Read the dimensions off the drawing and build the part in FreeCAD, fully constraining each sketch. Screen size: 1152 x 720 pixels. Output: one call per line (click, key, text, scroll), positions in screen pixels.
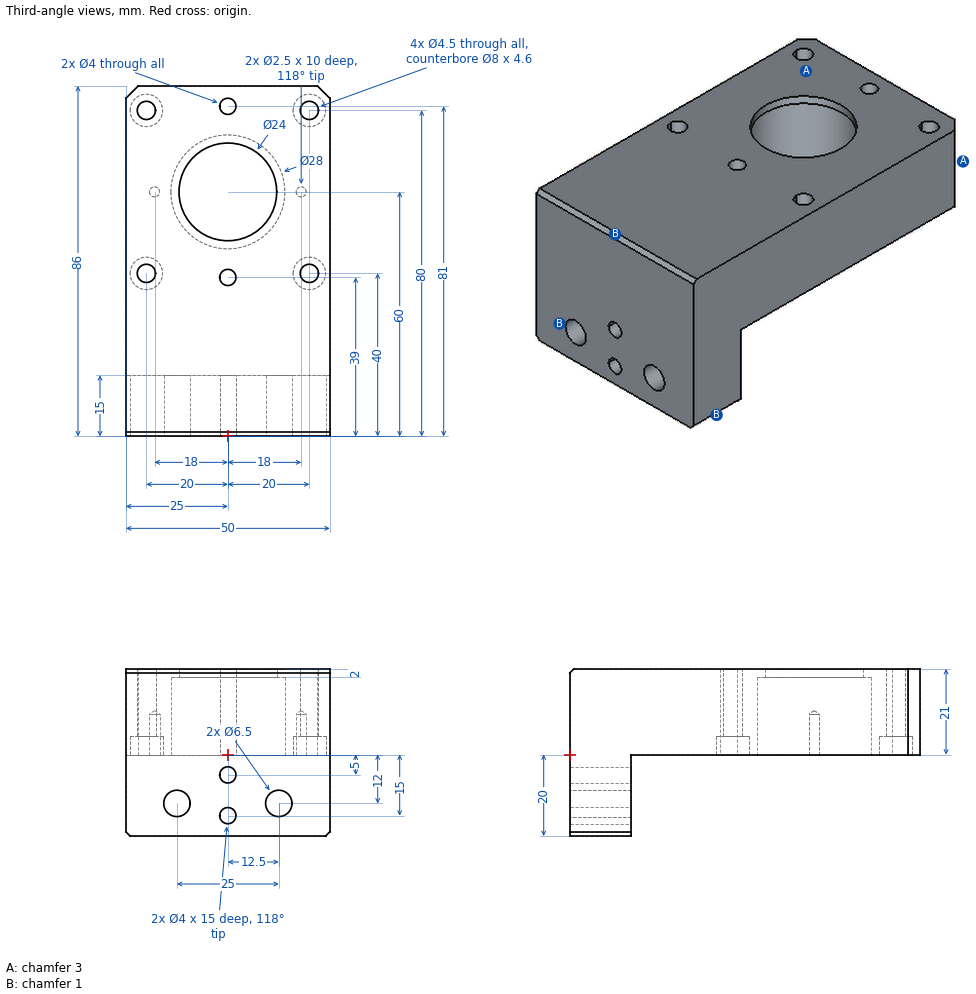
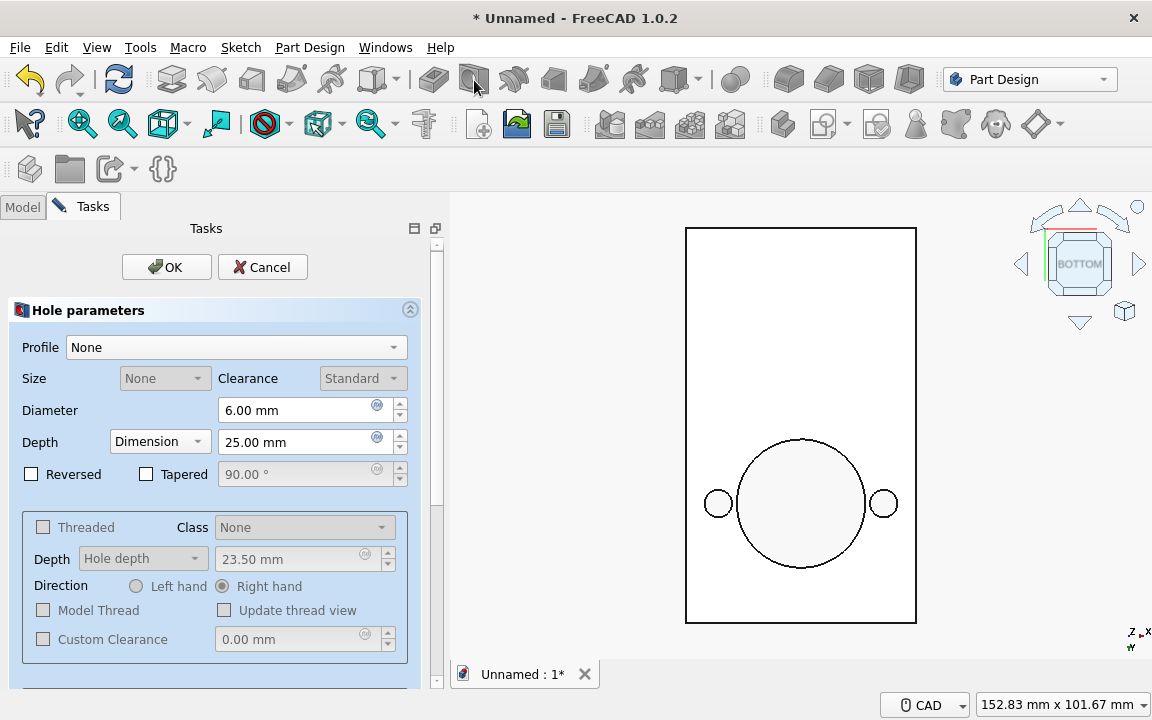
triple_click(305, 410)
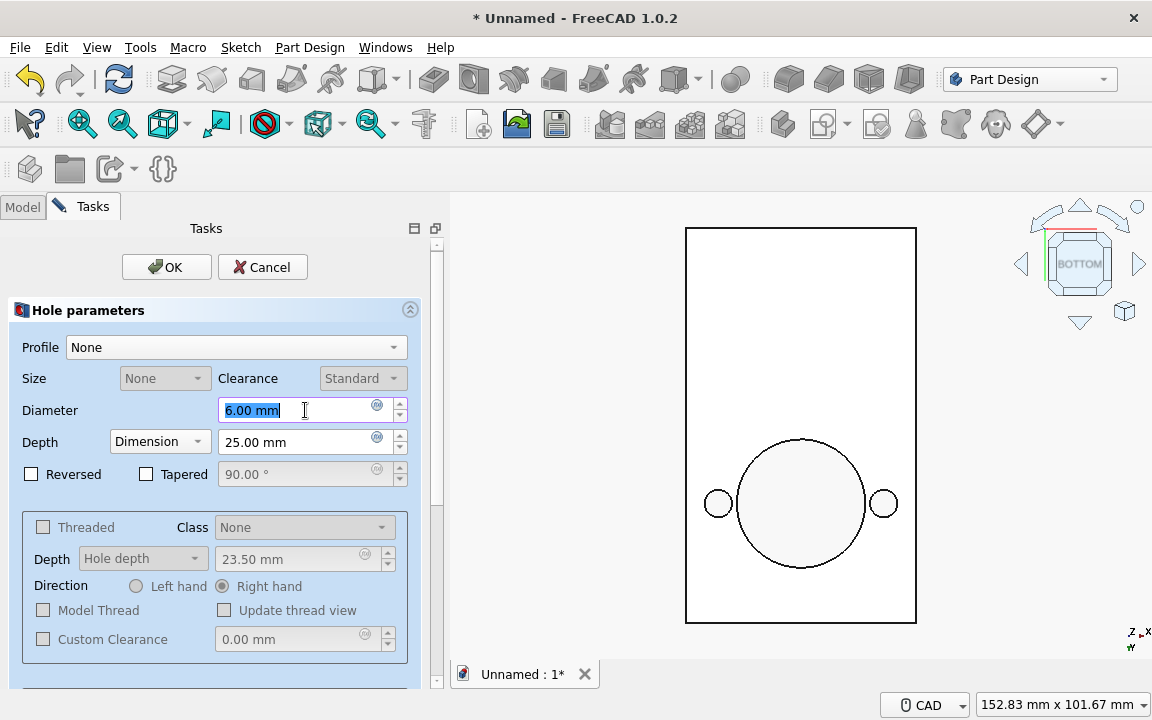
text(2.5)
key(Tab)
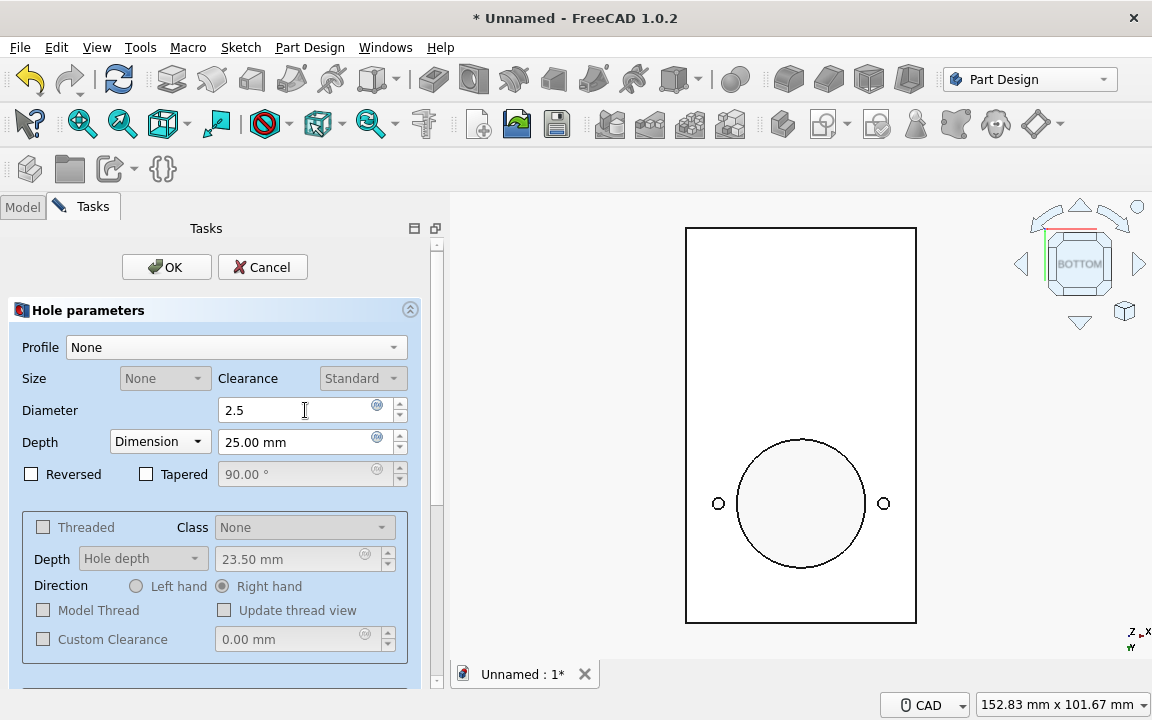
triple_click(305, 442)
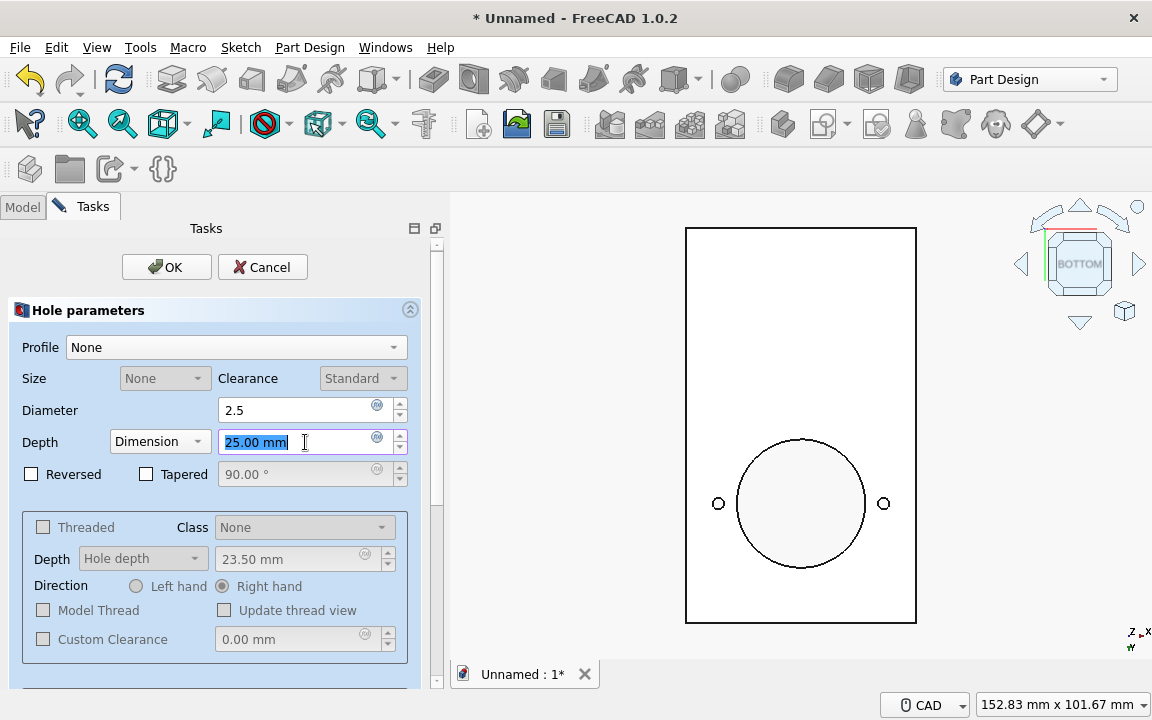
text(10)
key(Tab)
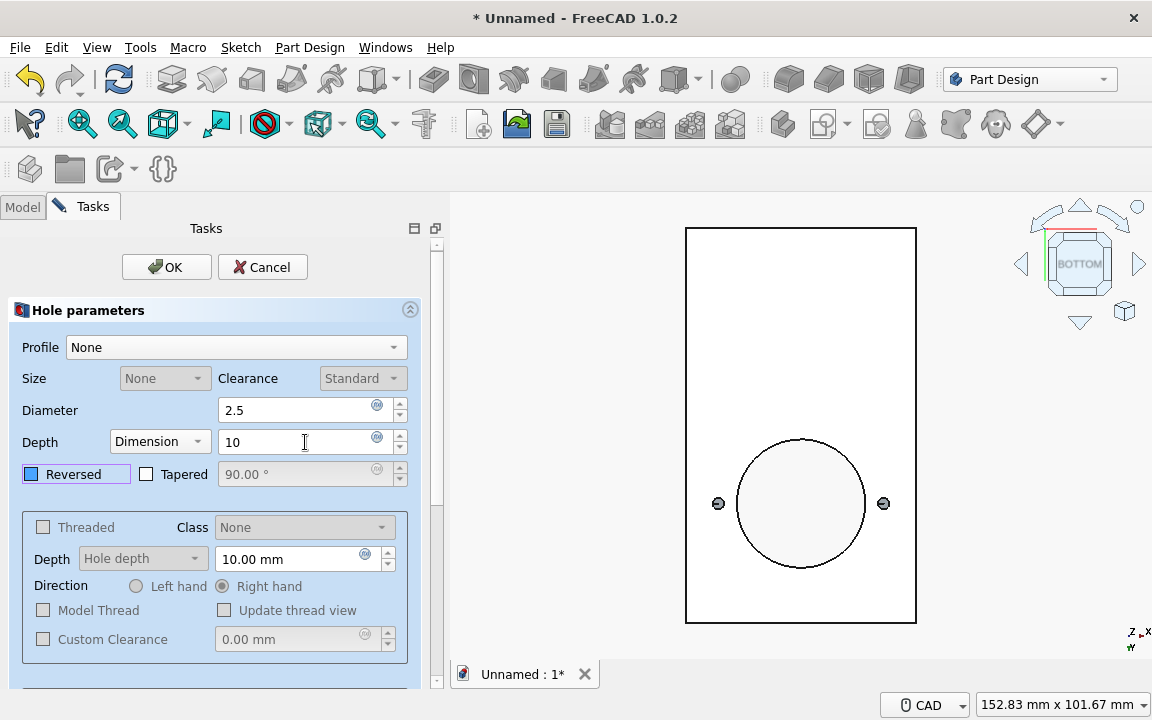
click(167, 267)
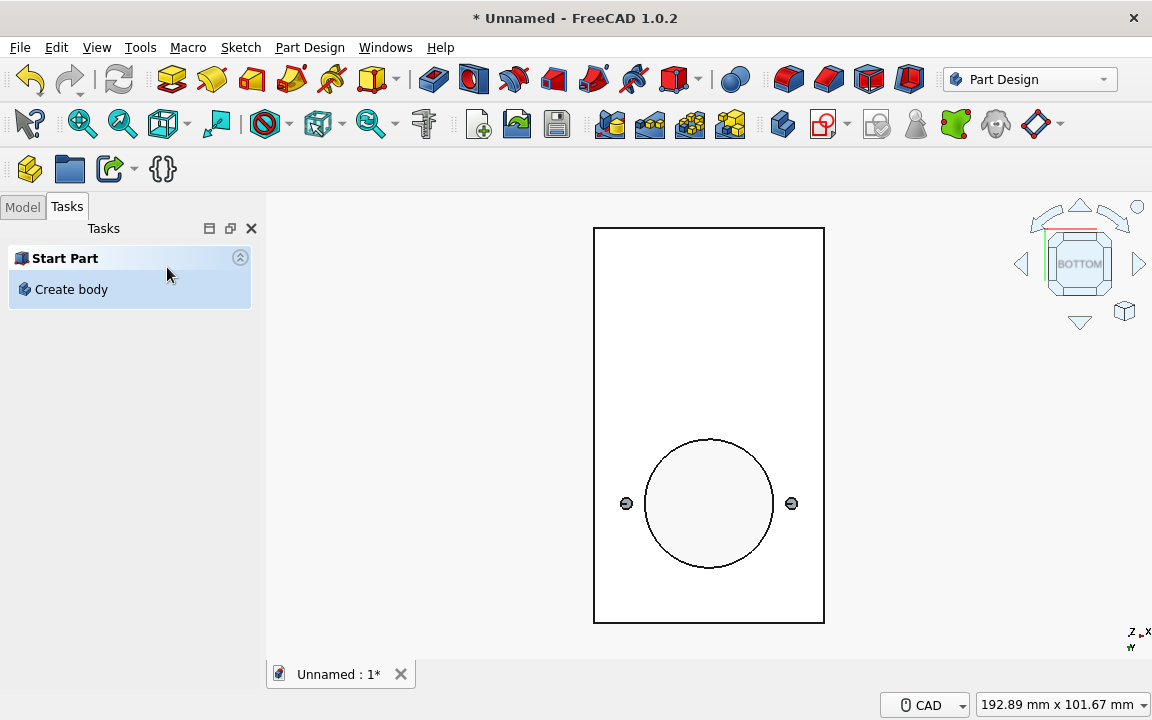
click(23, 206)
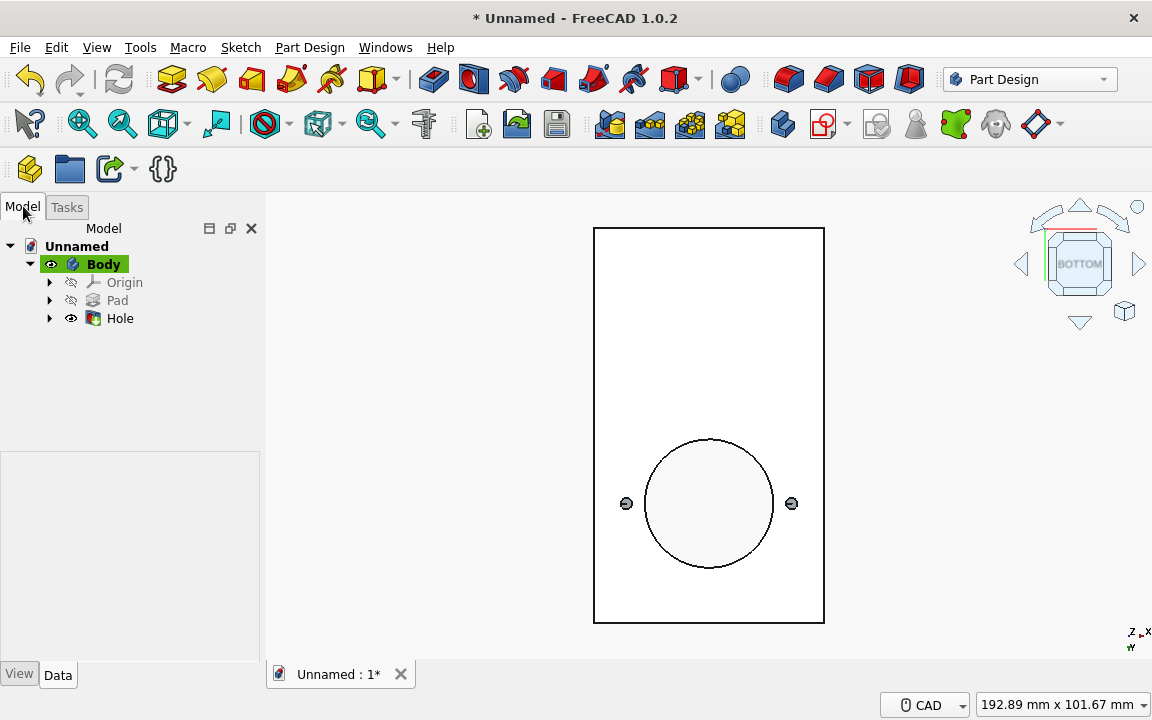
click(50, 282)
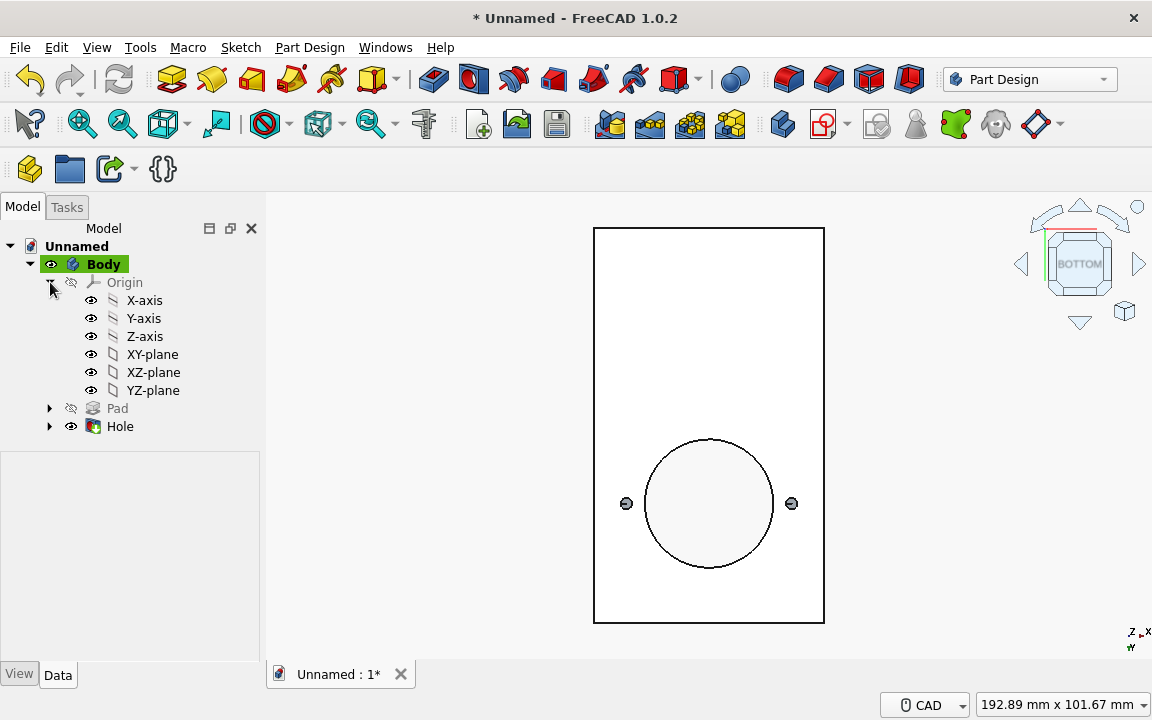
click(136, 354)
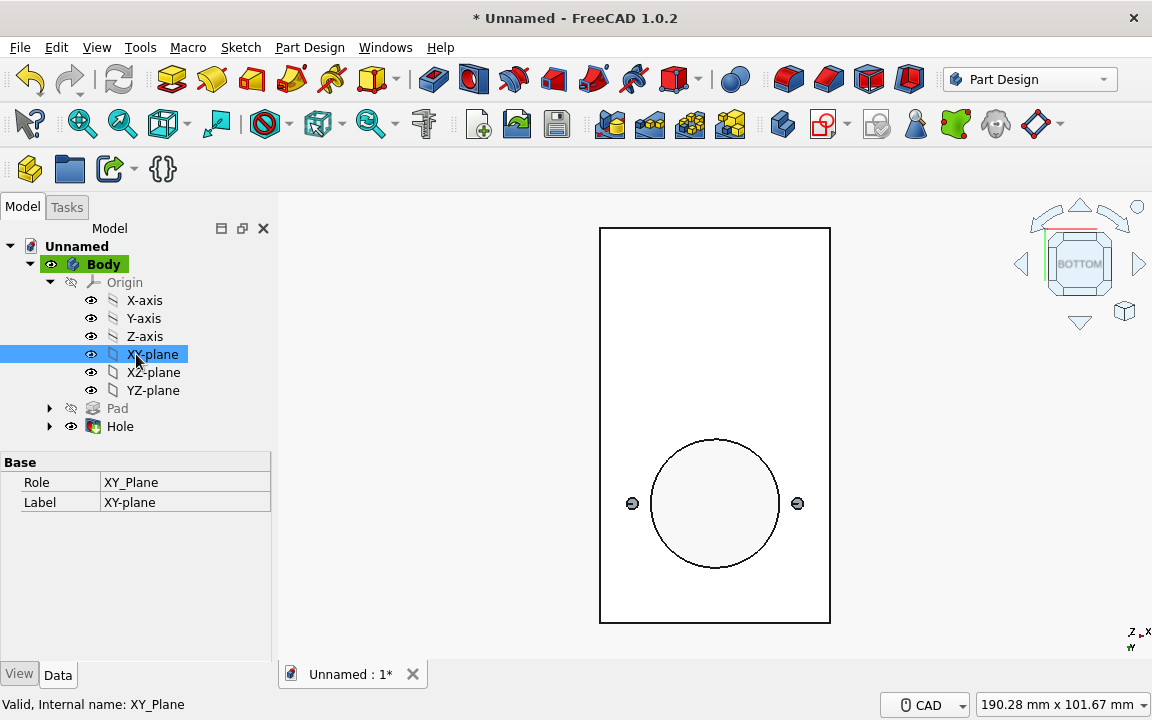
click(1036, 124)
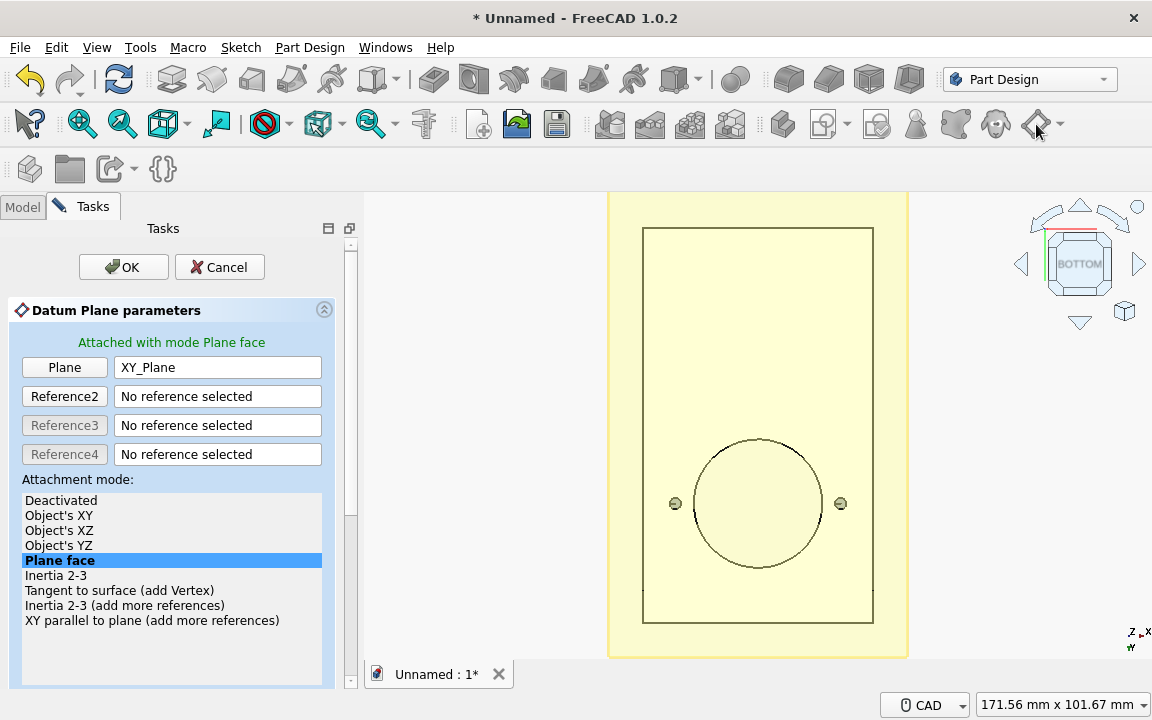
scroll(351, 463, down, 3)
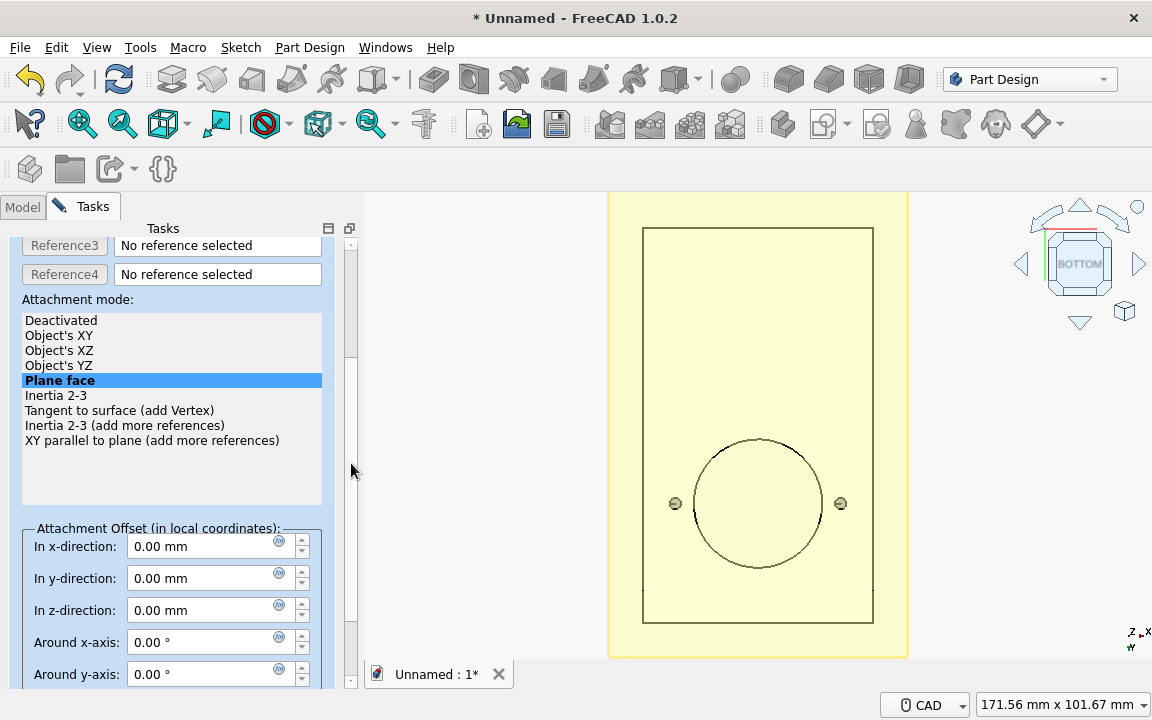
triple_click(210, 610)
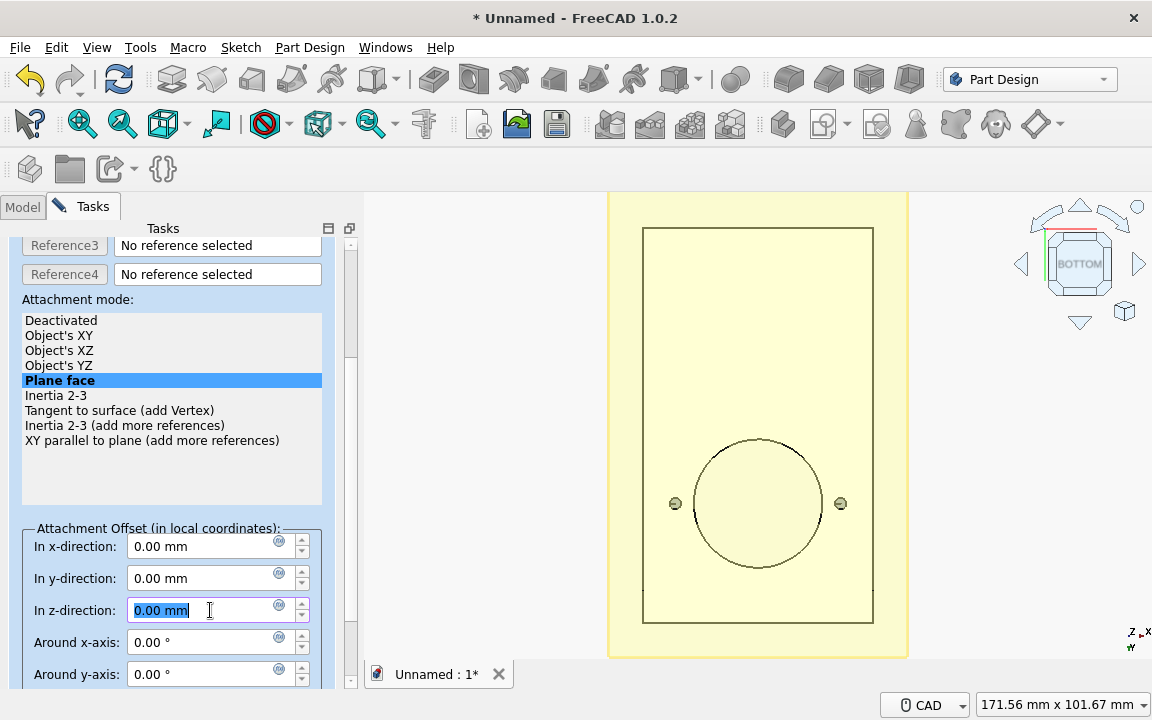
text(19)
key(Tab)